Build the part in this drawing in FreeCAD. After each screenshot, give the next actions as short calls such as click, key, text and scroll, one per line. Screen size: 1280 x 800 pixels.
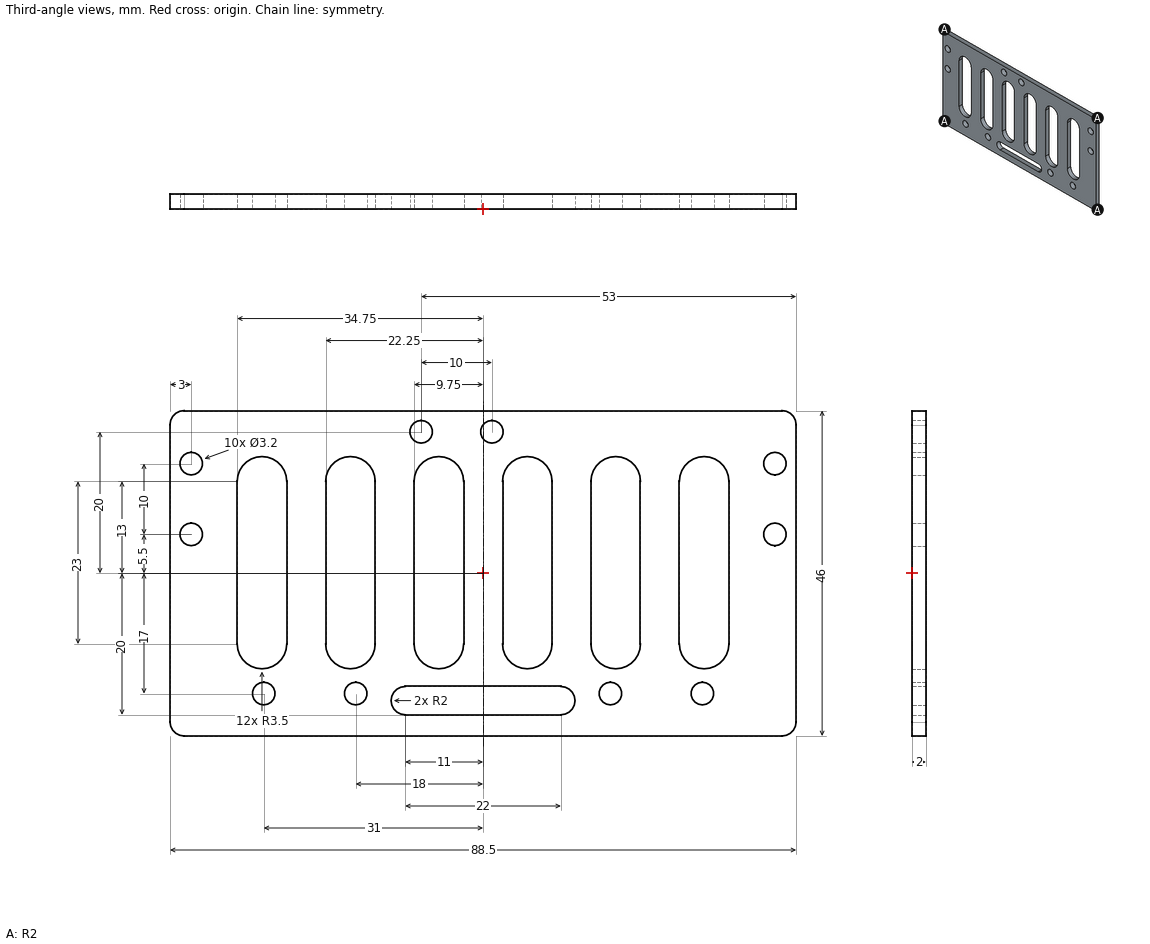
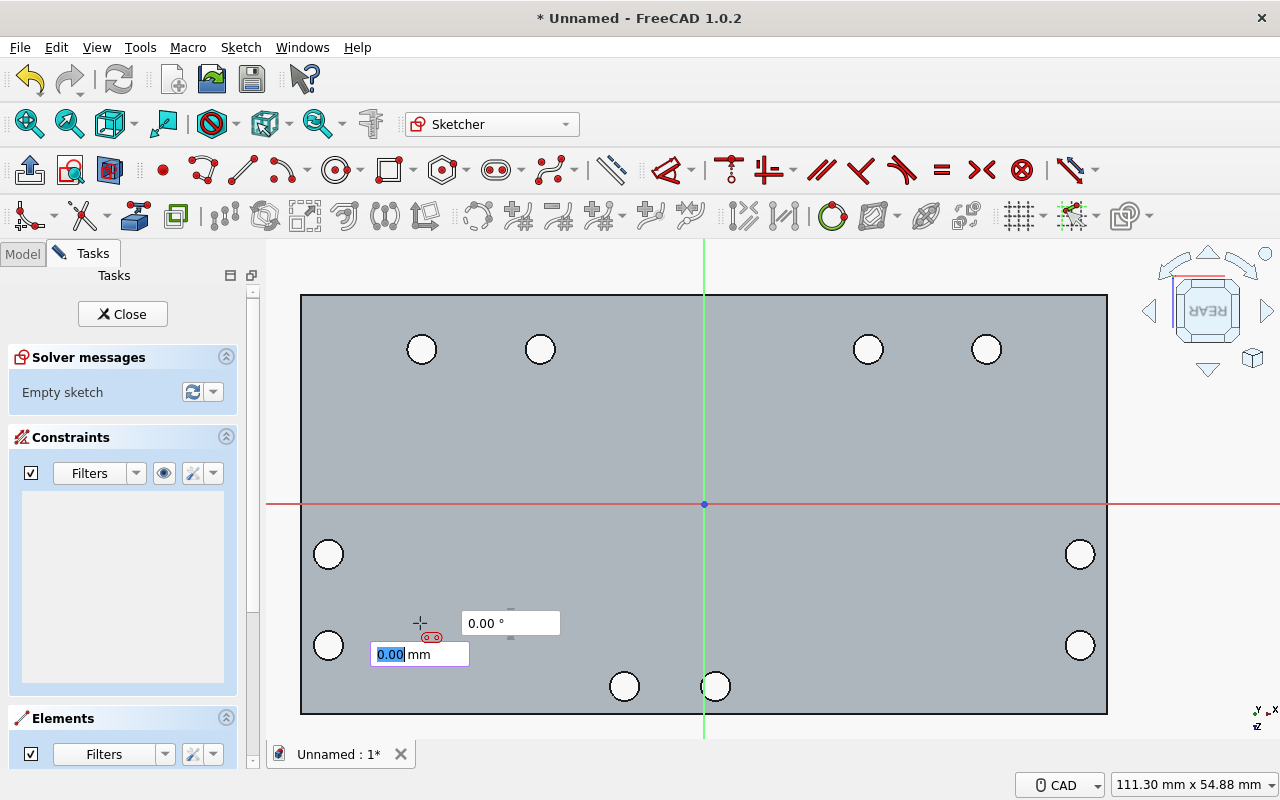
click(420, 413)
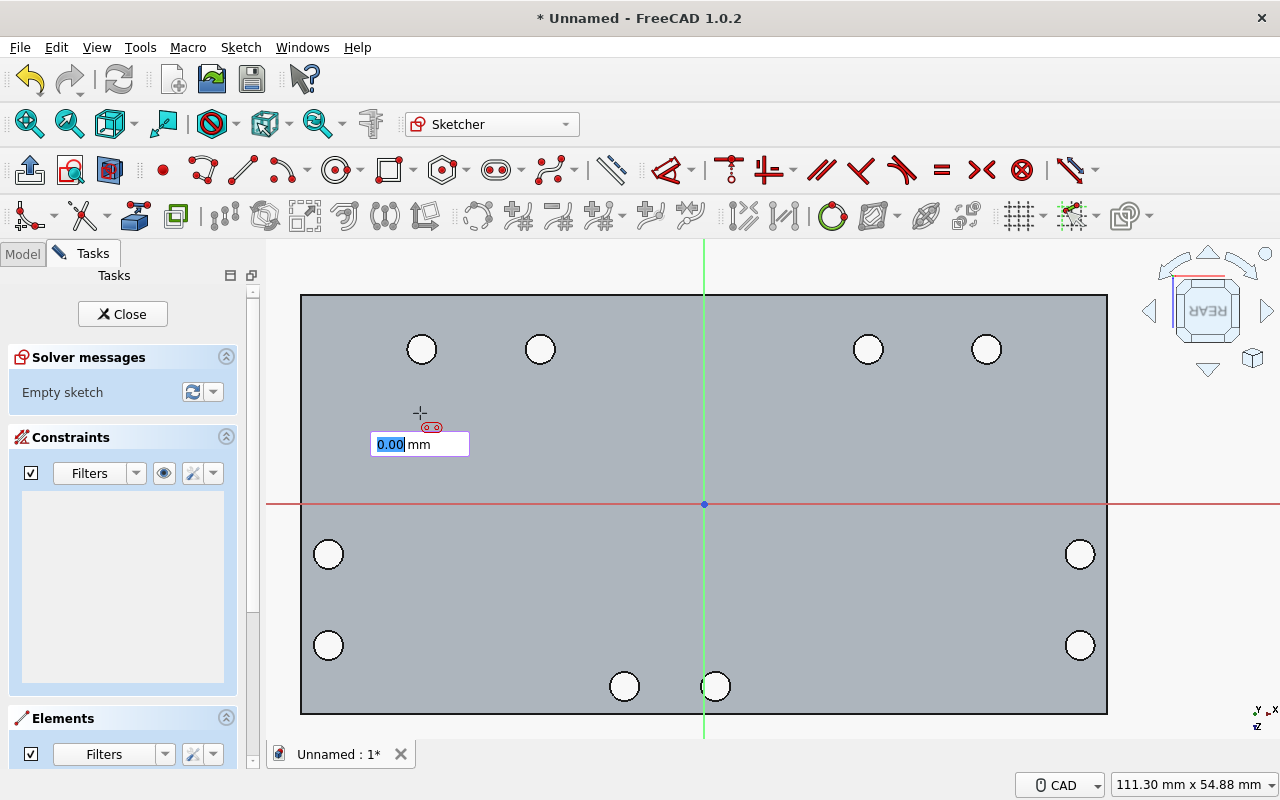
click(451, 549)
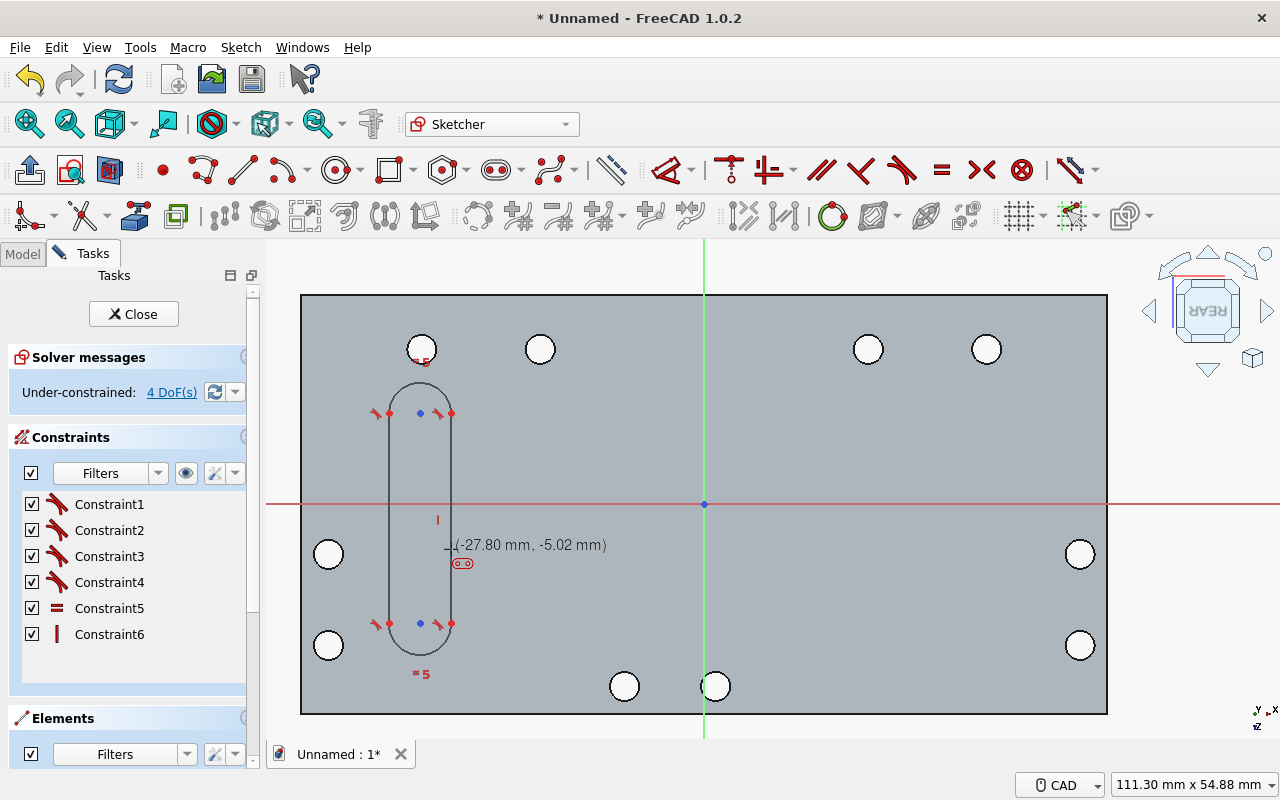
click(533, 623)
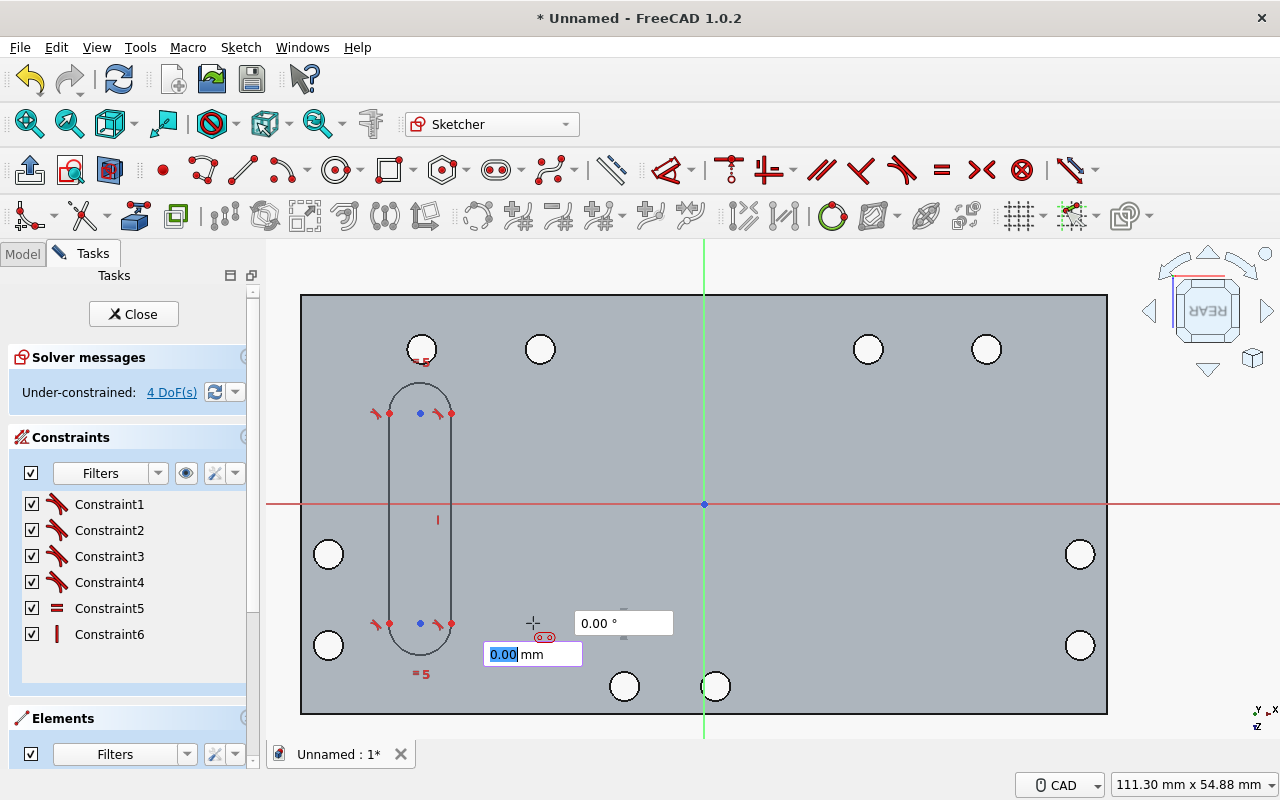
click(533, 413)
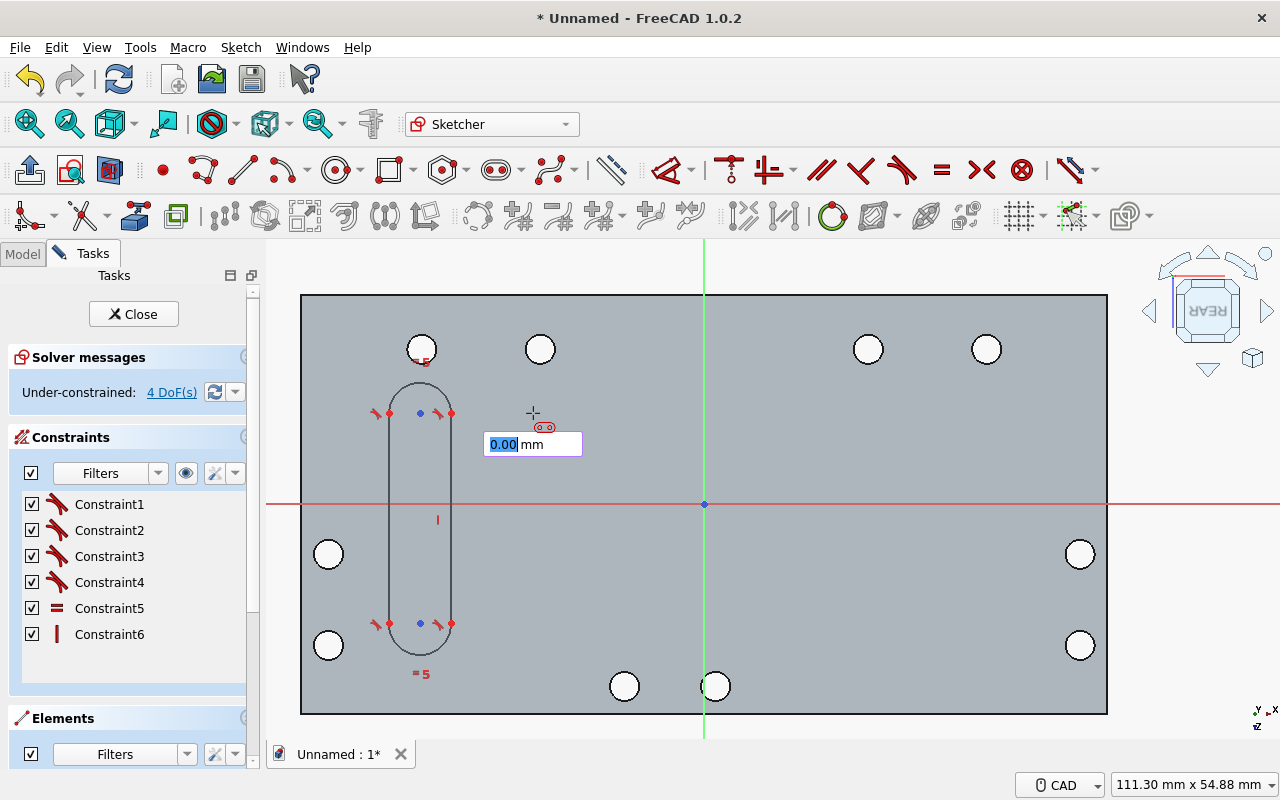
click(565, 549)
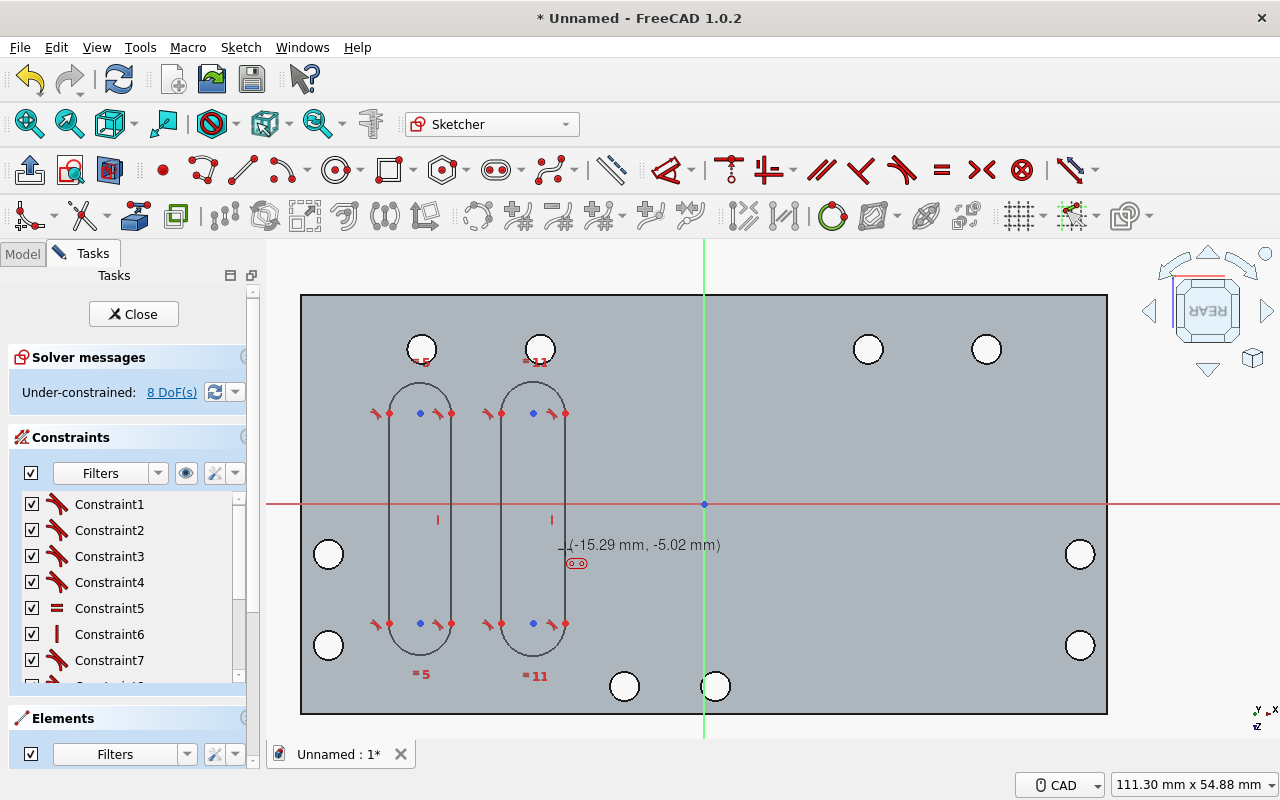
click(647, 623)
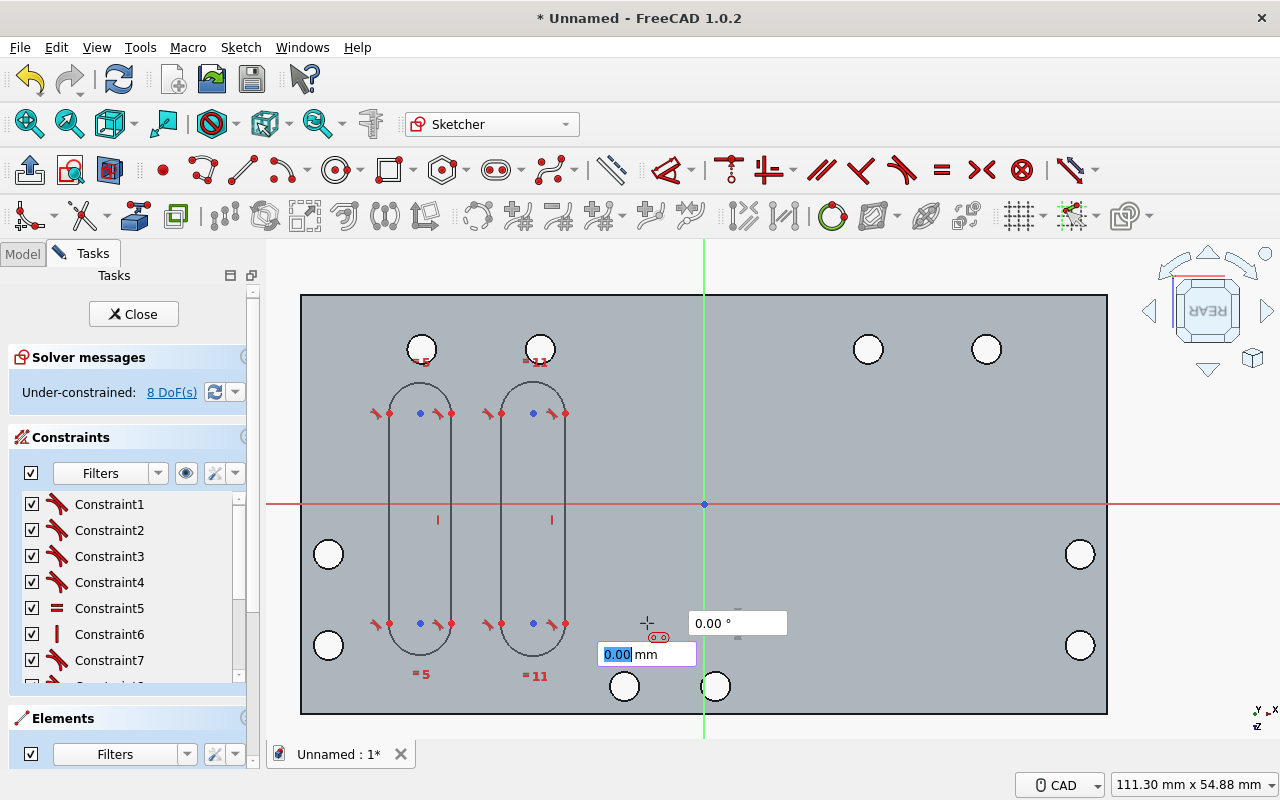
click(647, 413)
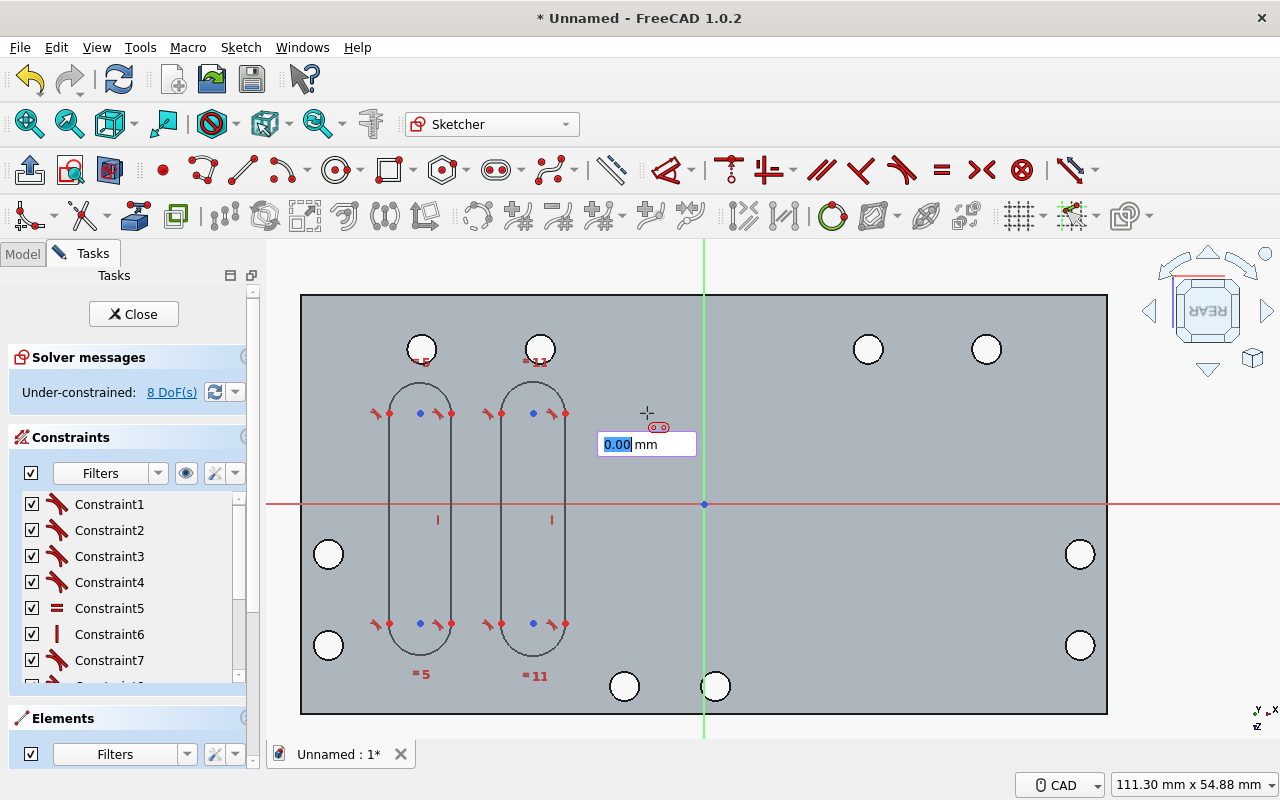
click(679, 549)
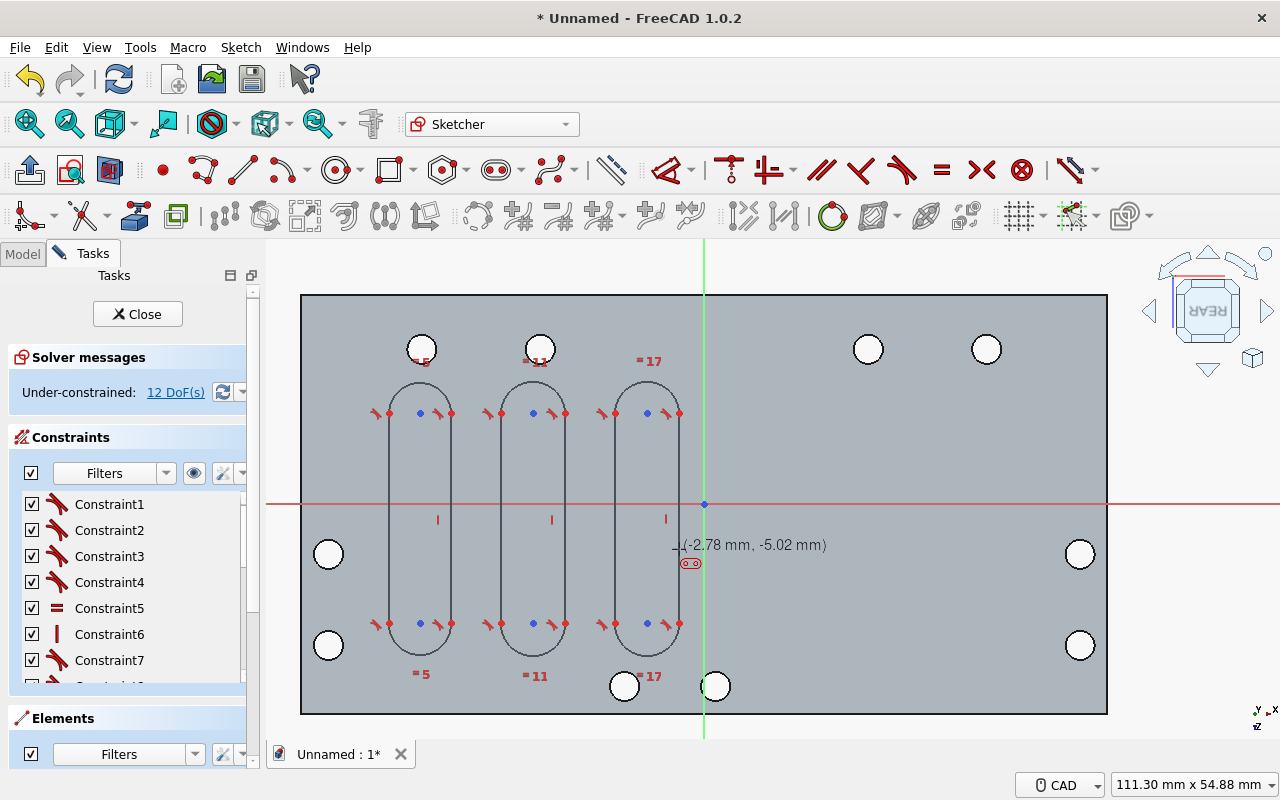
click(761, 623)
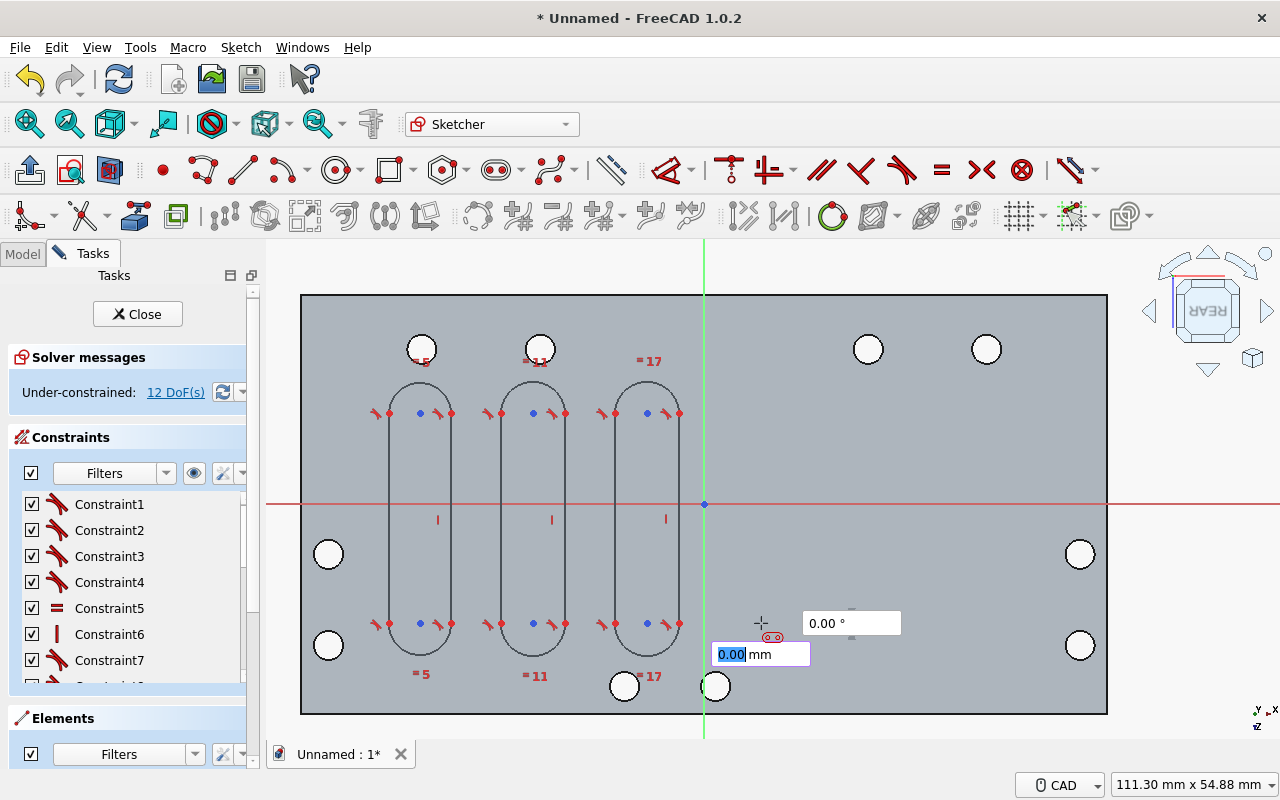
click(761, 413)